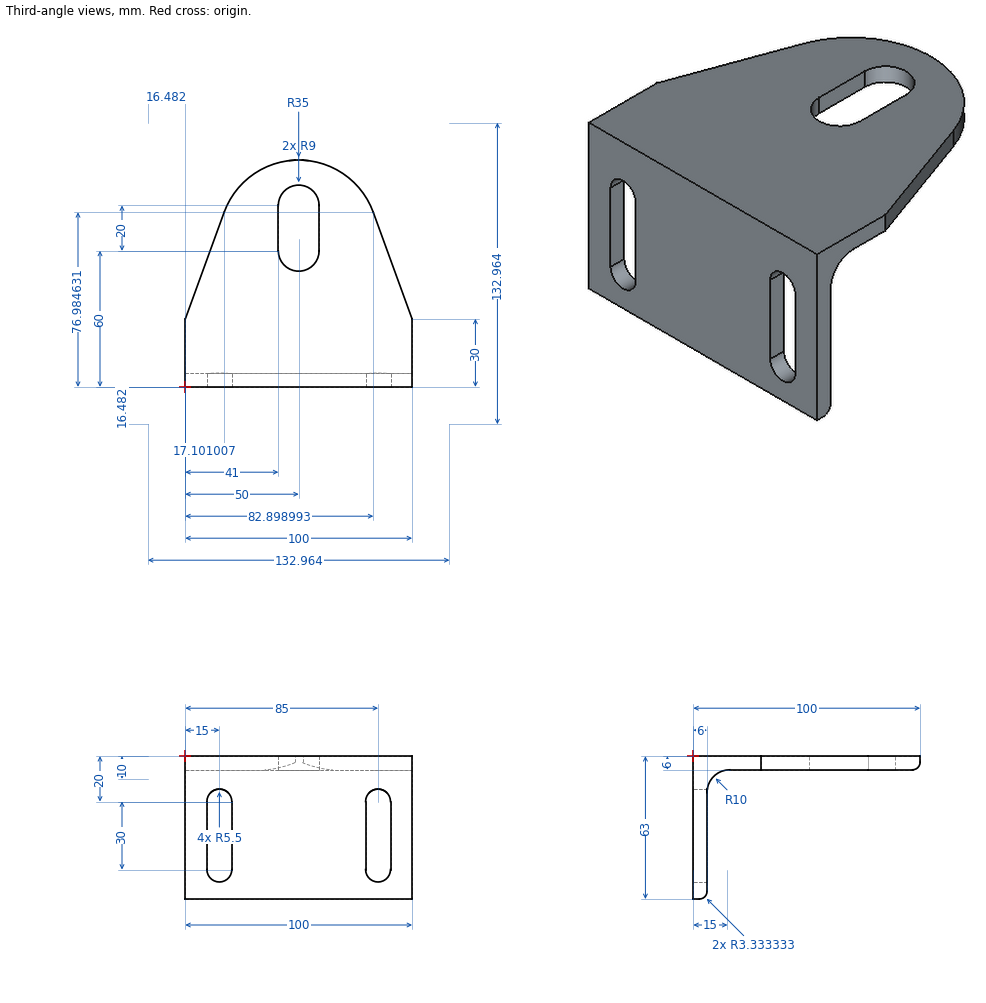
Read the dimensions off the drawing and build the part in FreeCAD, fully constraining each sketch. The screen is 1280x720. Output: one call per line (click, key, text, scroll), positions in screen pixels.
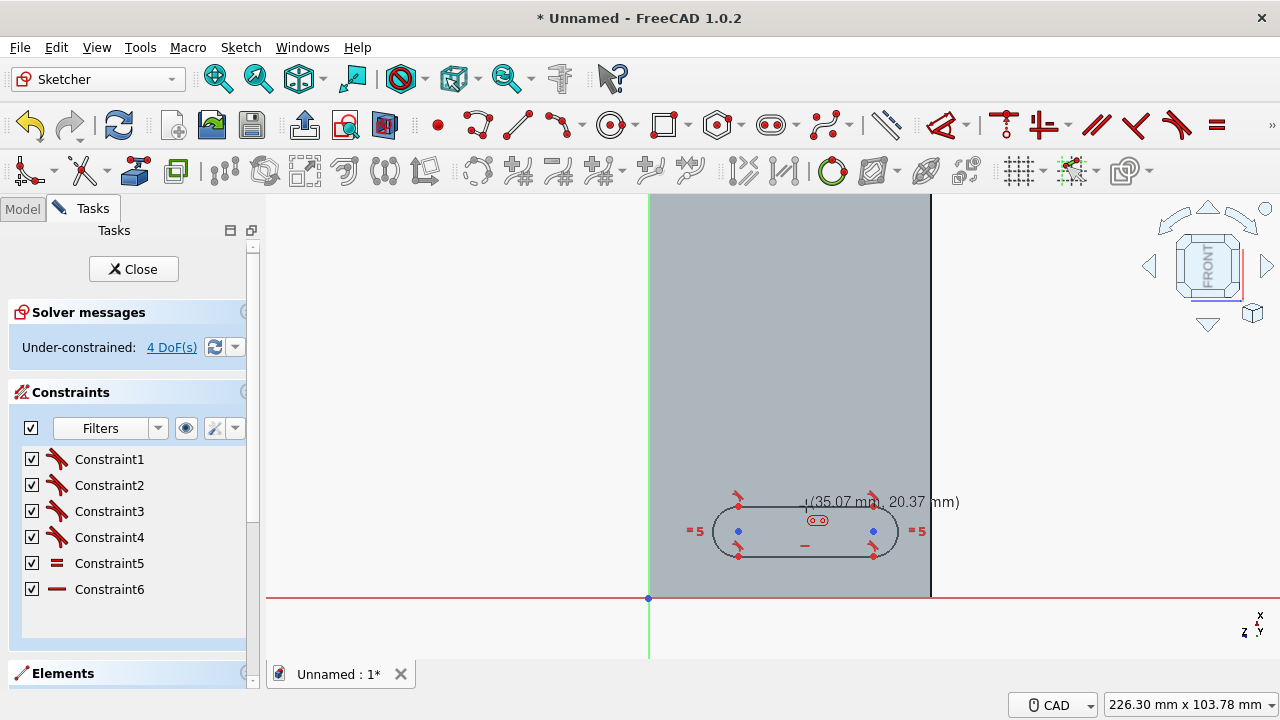
scroll(565, 489, down, 2)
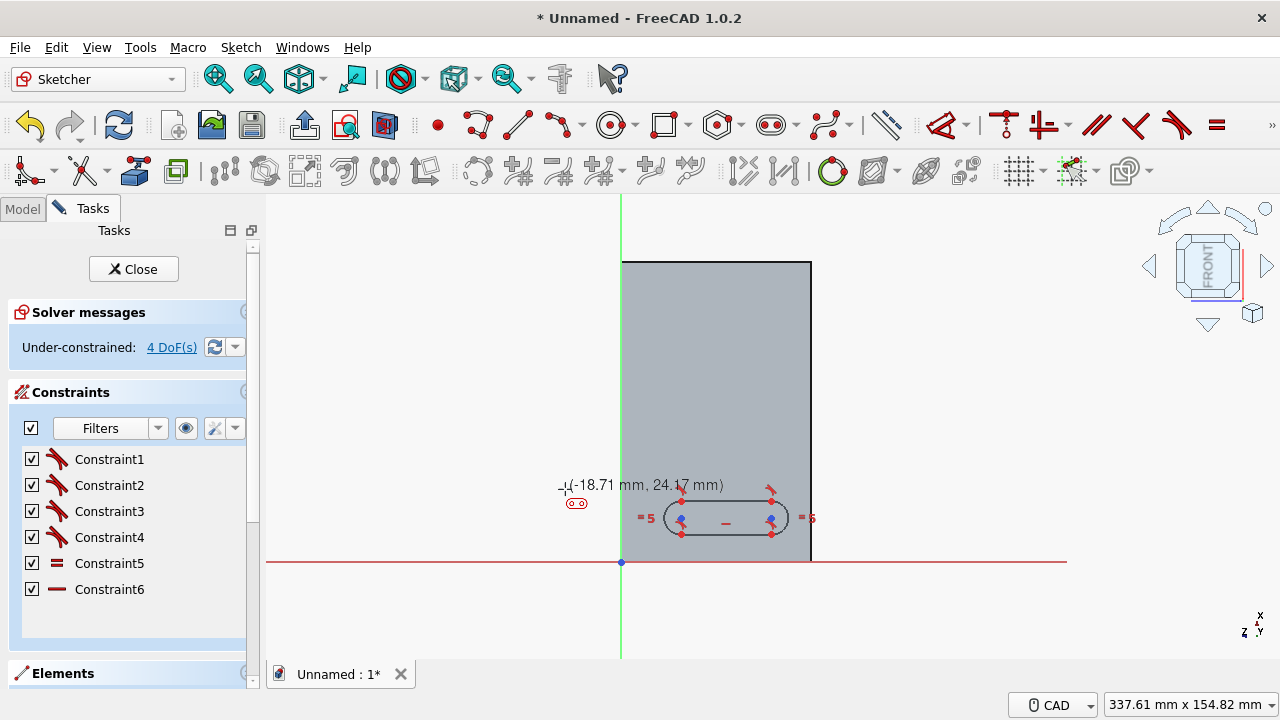
scroll(681, 307, up, 2)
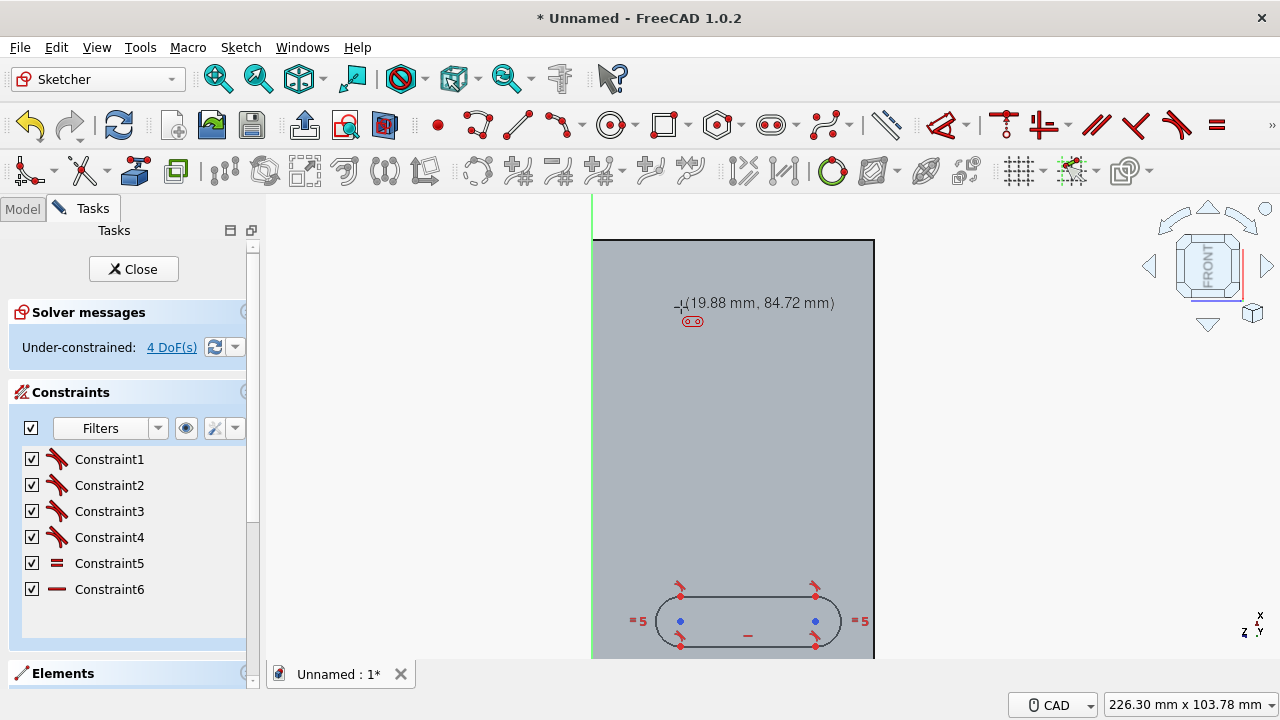
click(681, 307)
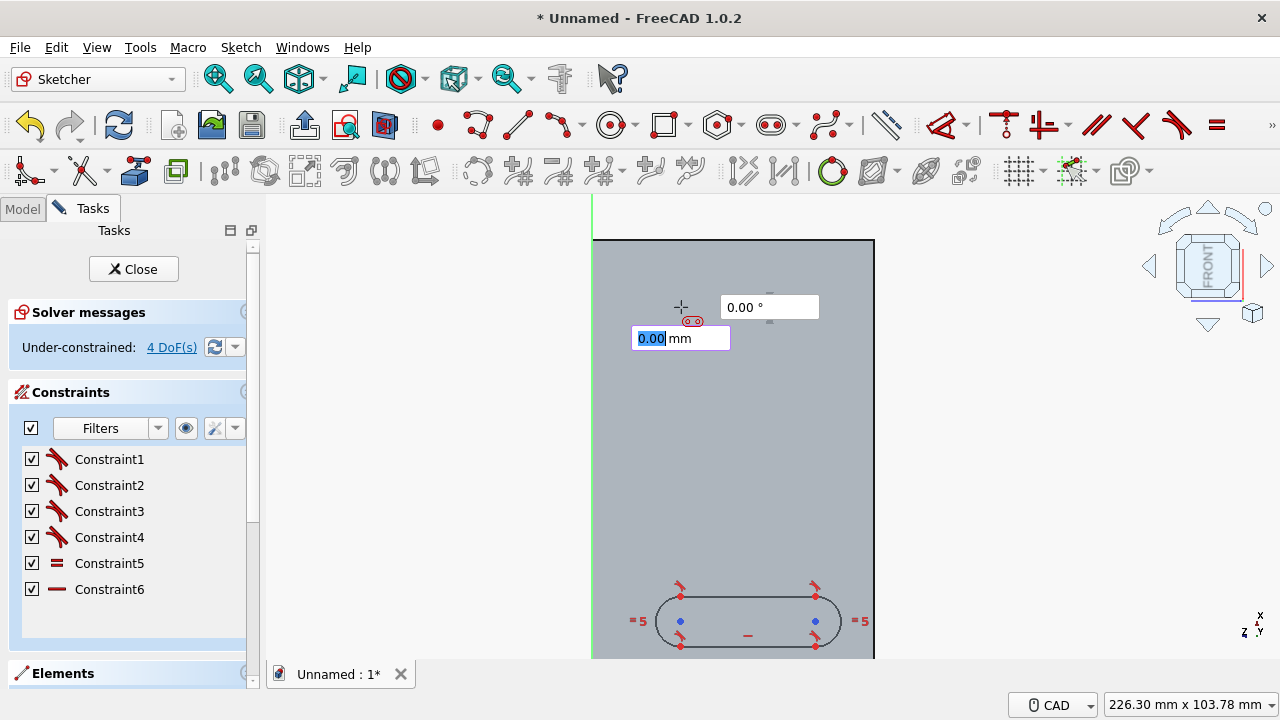
click(816, 307)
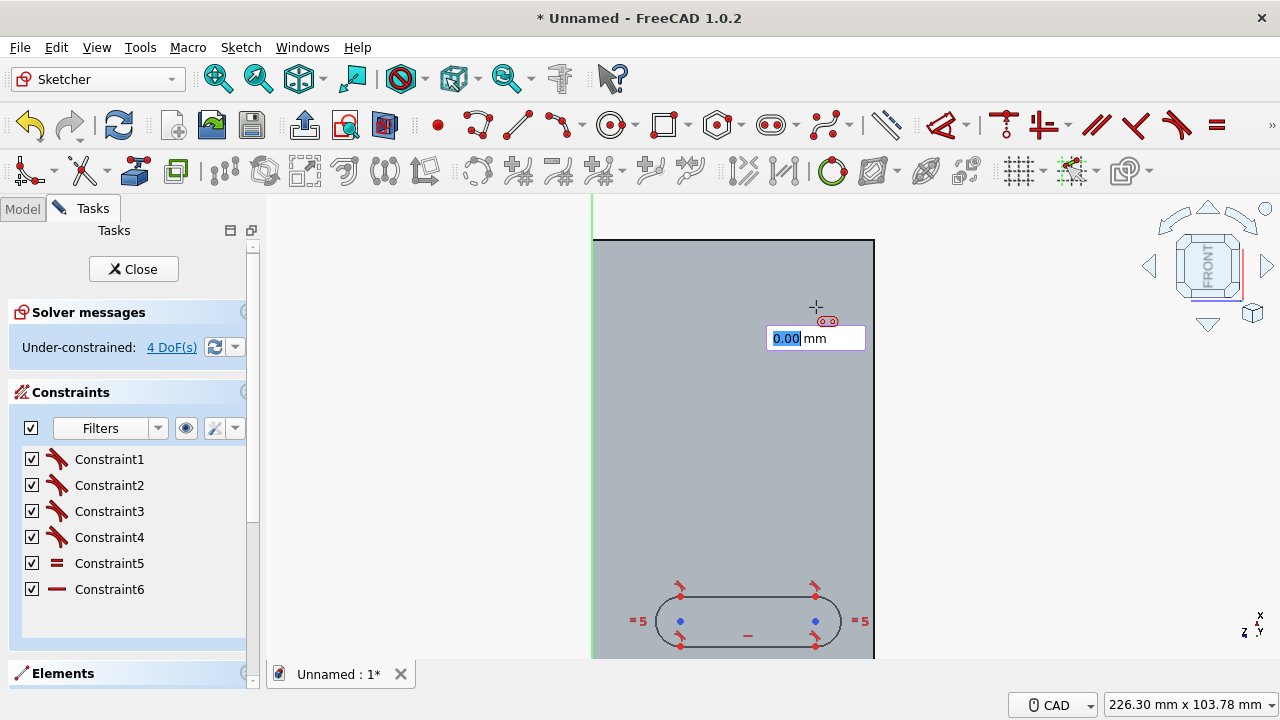
click(749, 332)
key(Escape)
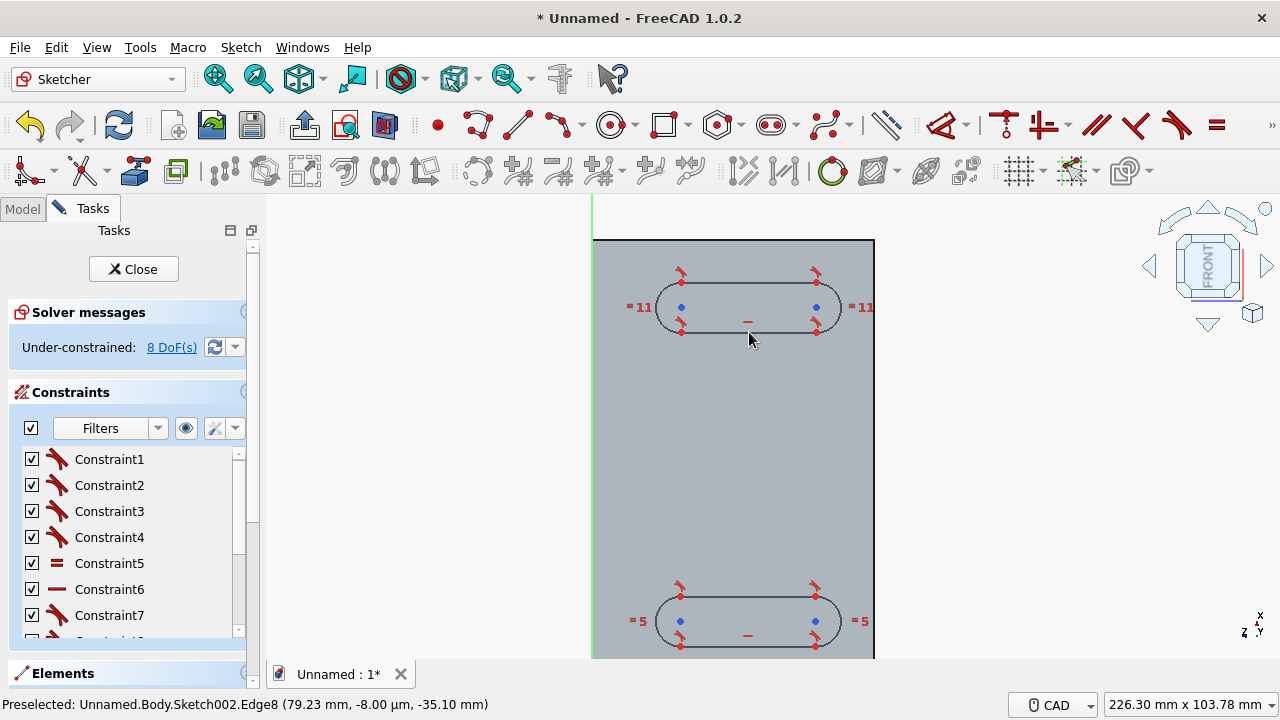
click(661, 607)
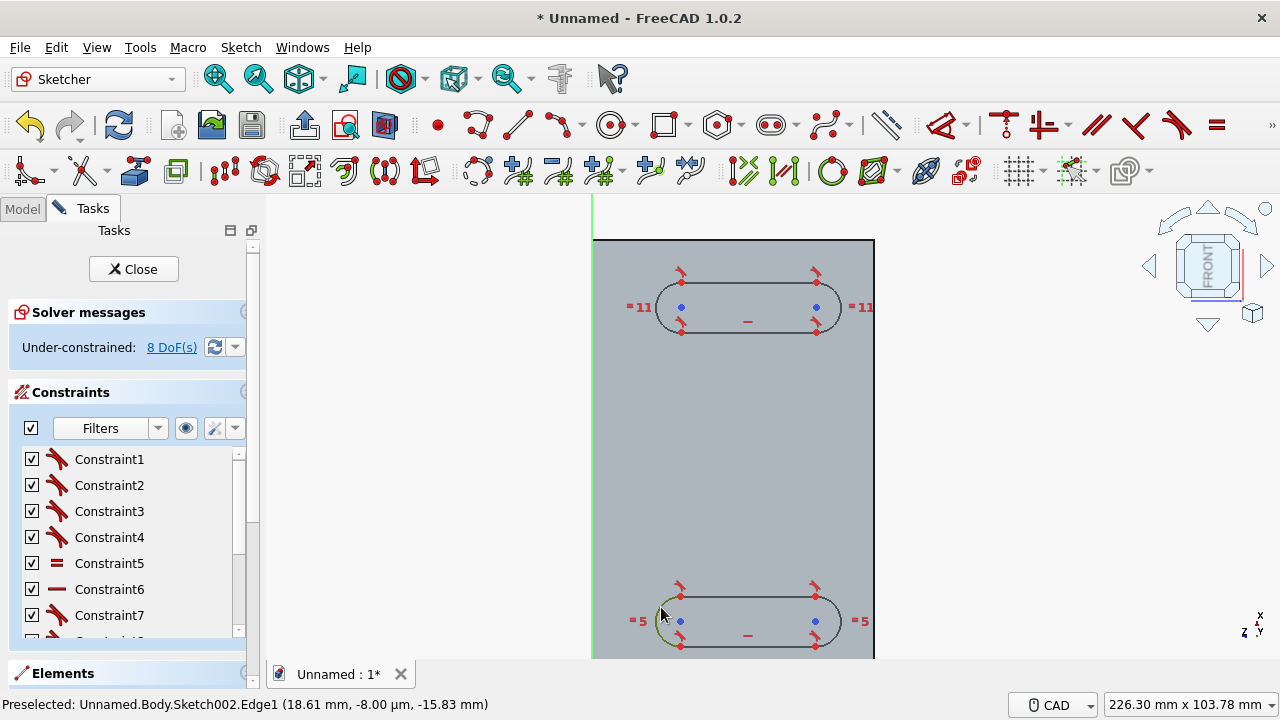
click(661, 293)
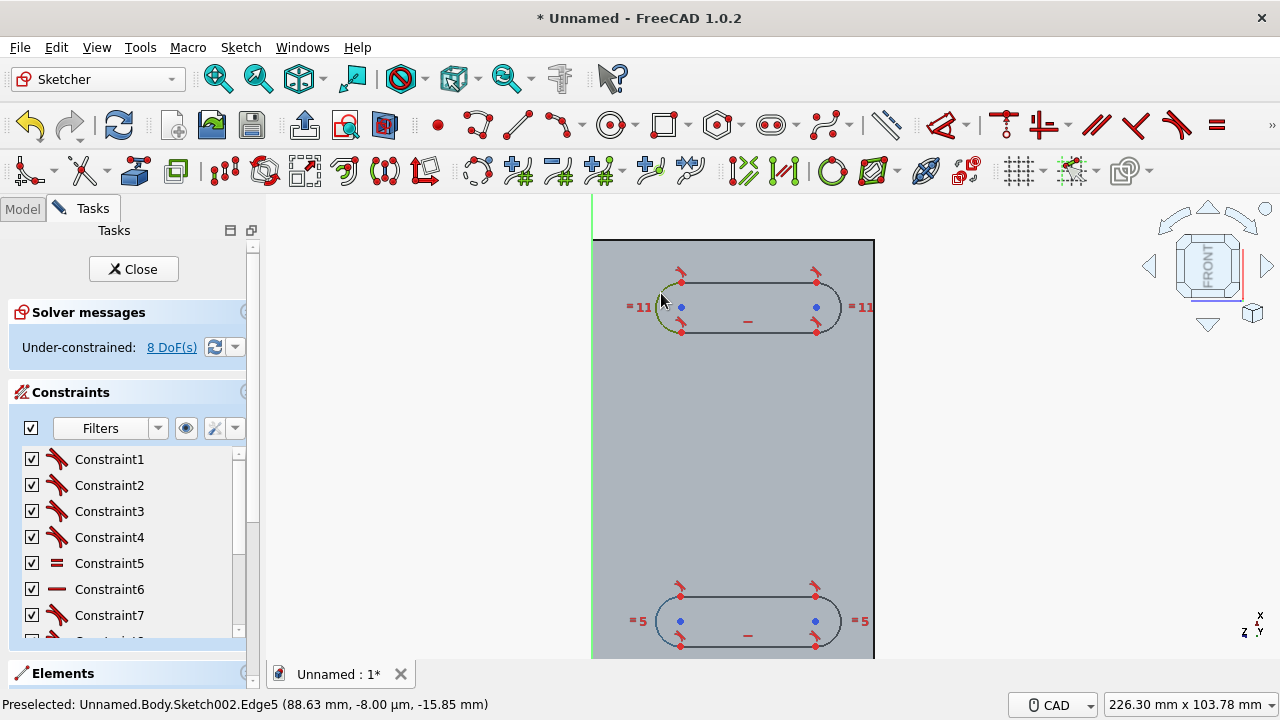
click(1218, 126)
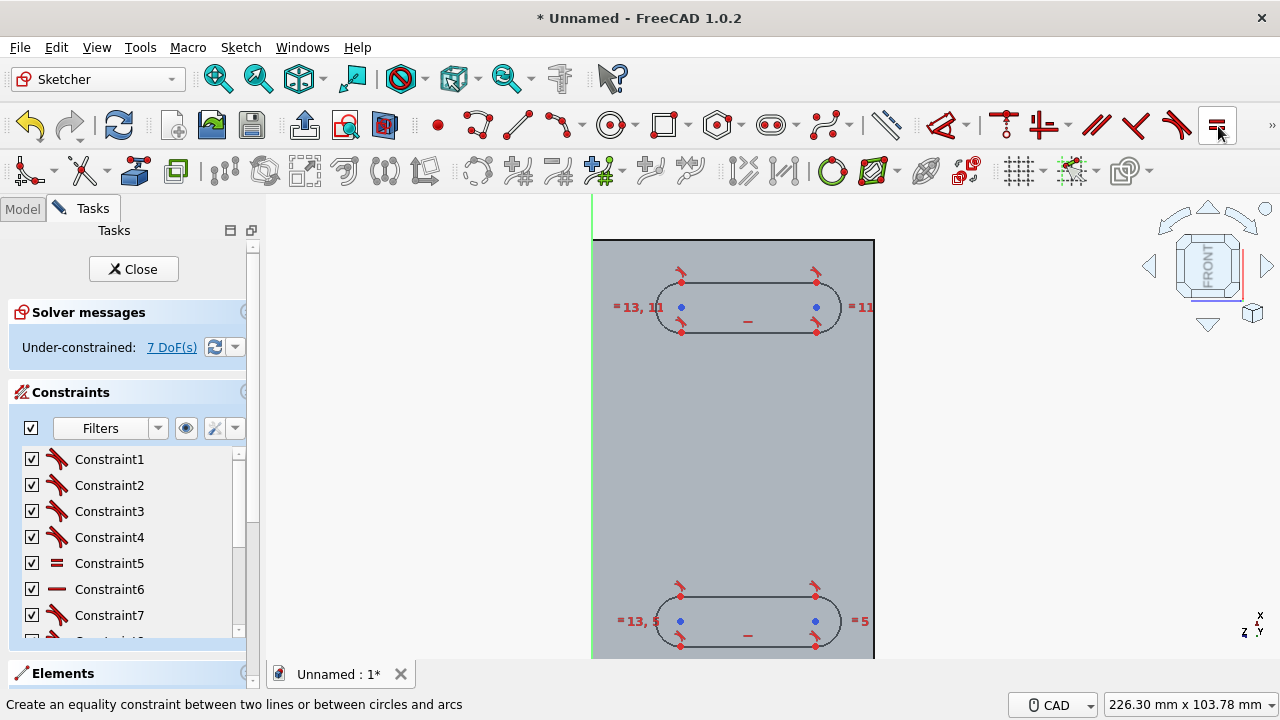
scroll(661, 607, up, 3)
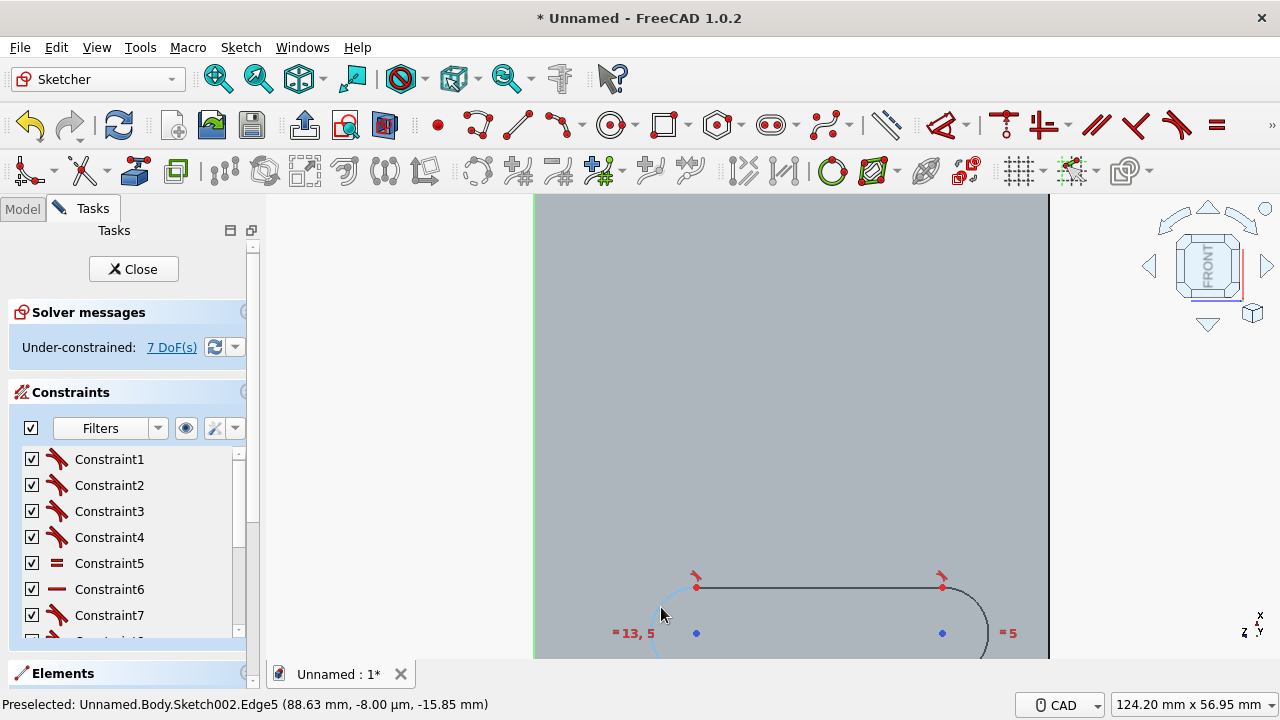
click(660, 606)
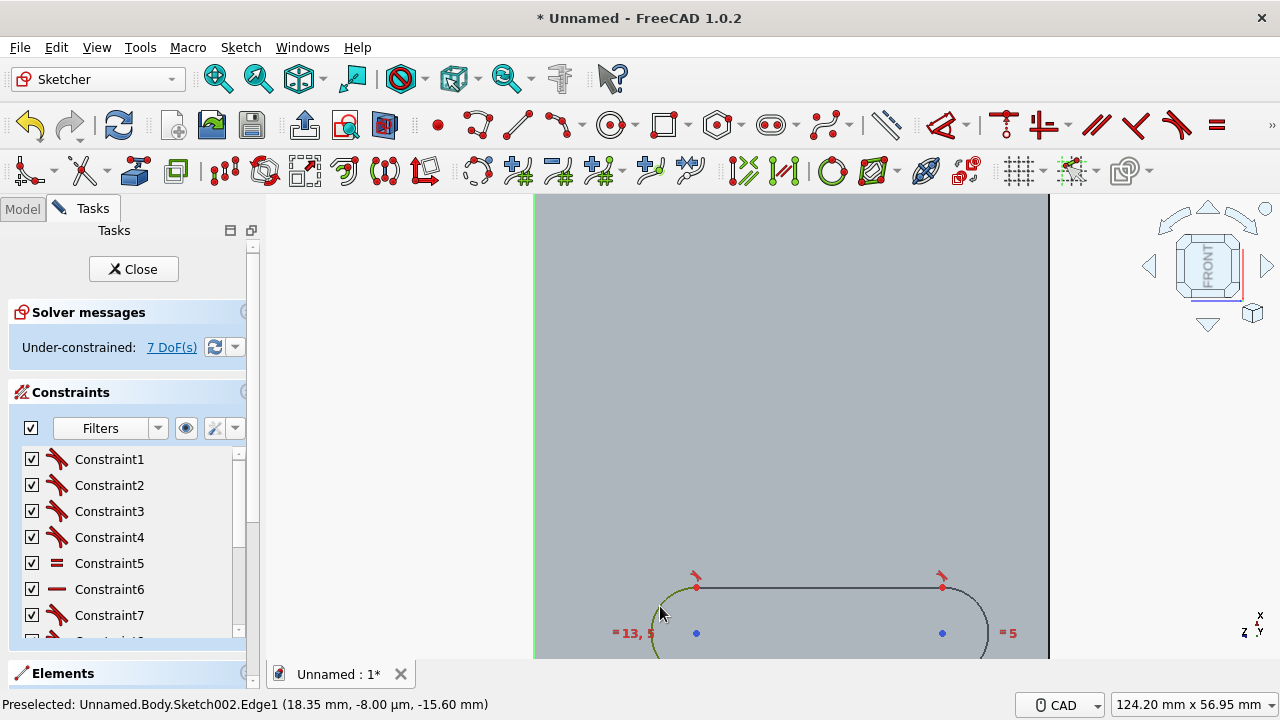
key(k)
key(r)